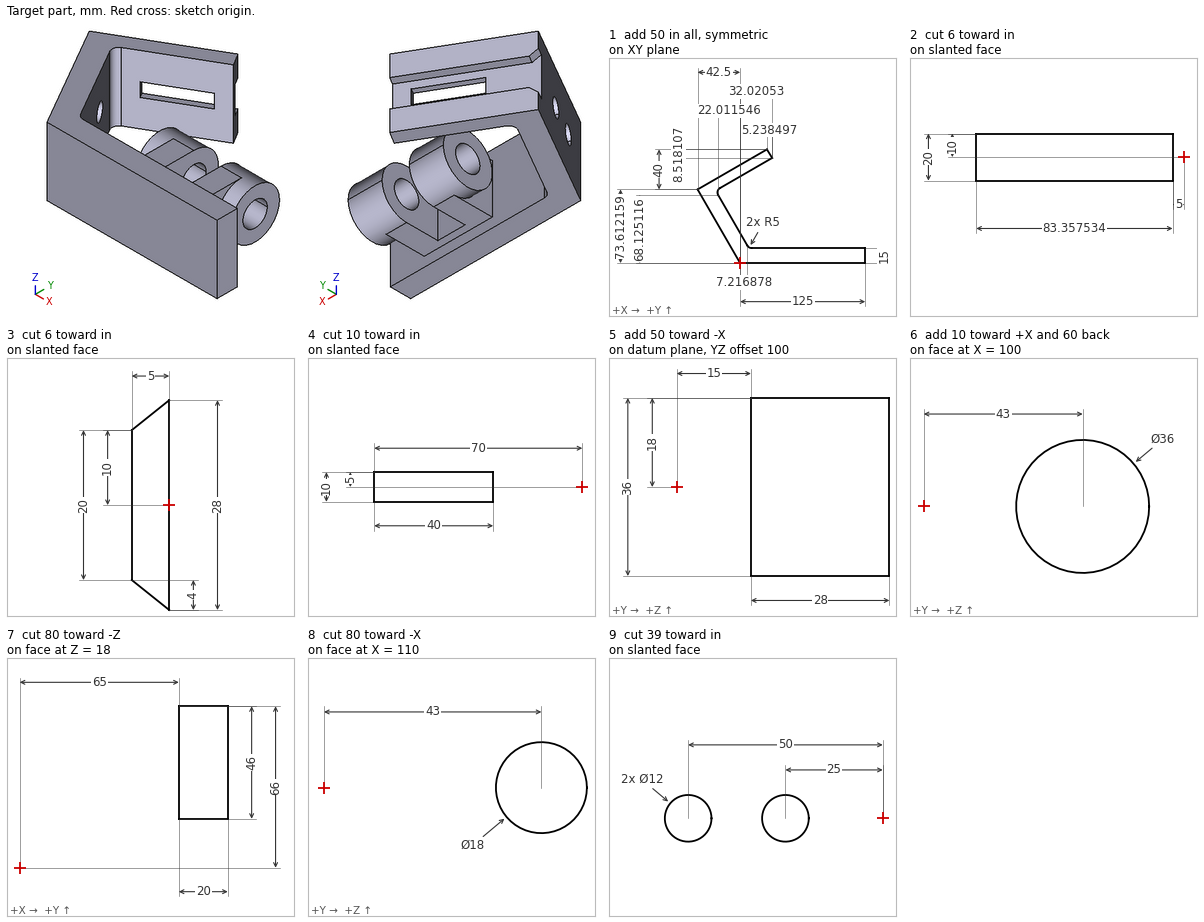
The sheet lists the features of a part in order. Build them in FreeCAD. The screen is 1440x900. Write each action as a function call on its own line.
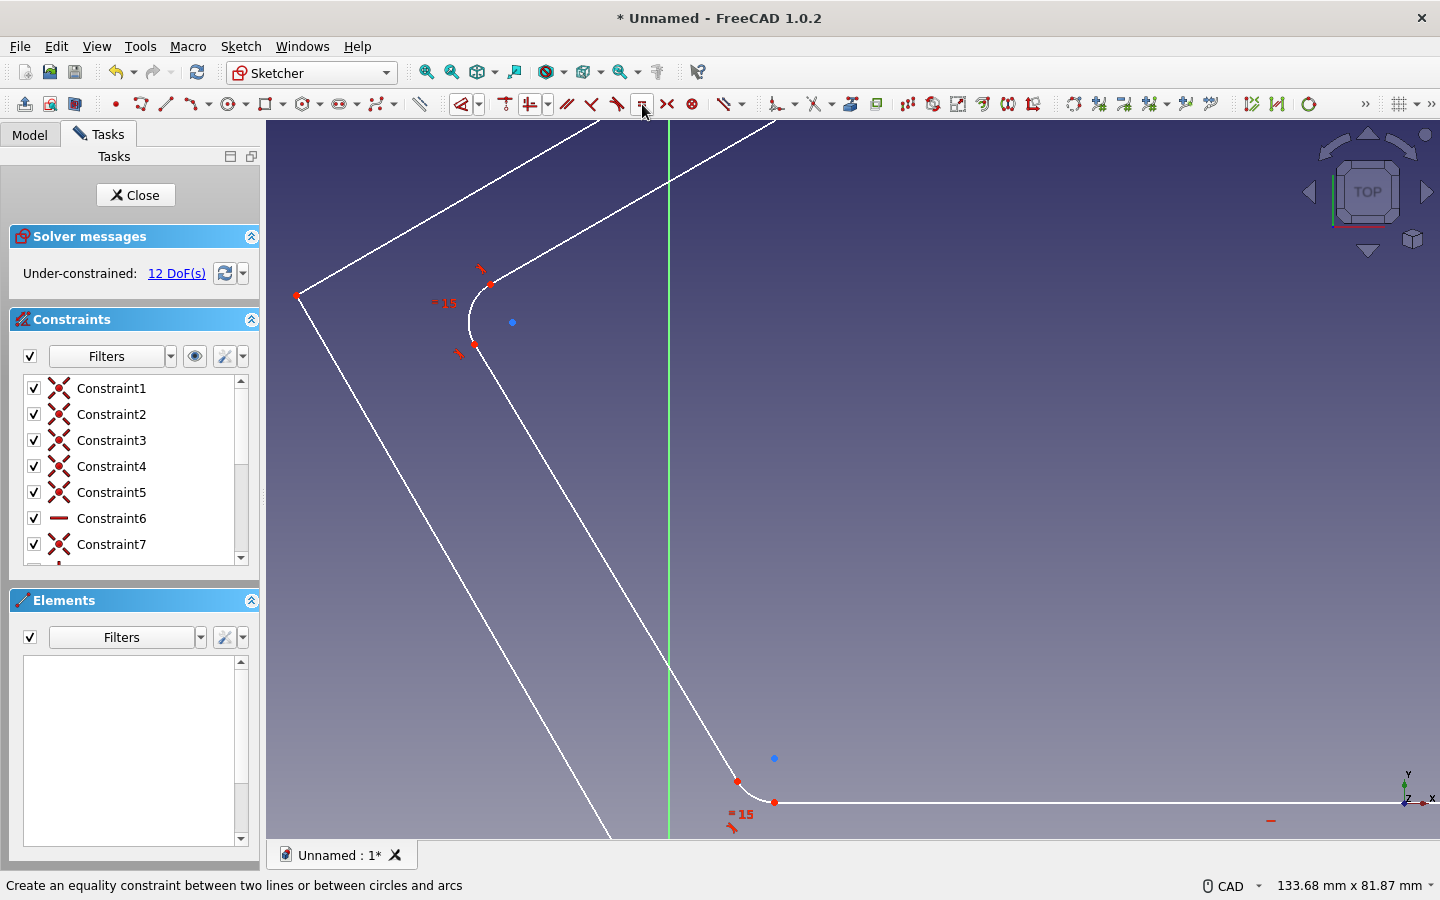
click(460, 104)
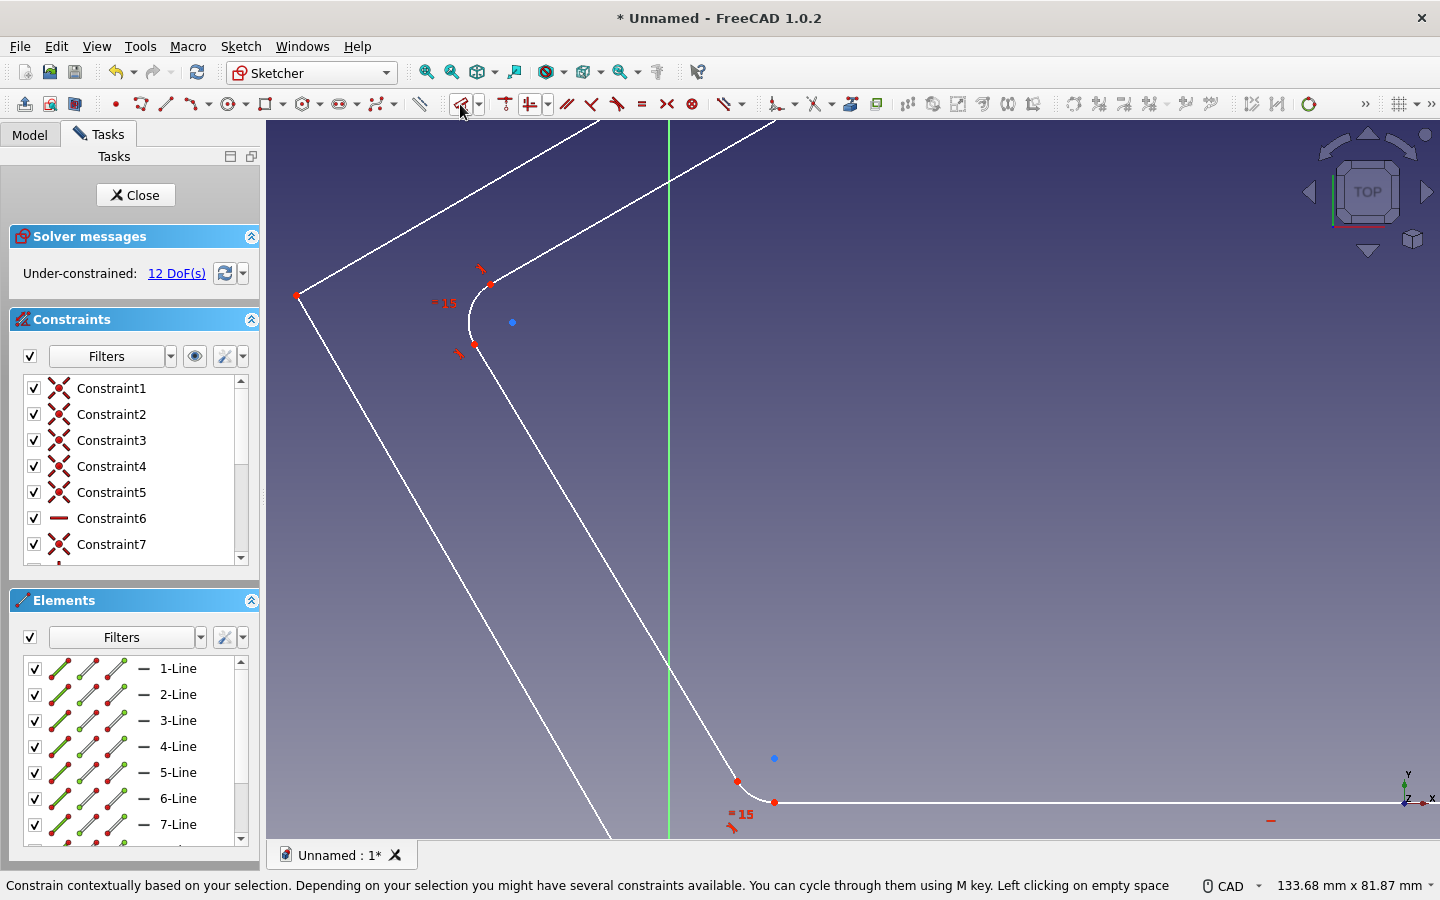
click(476, 299)
click(449, 282)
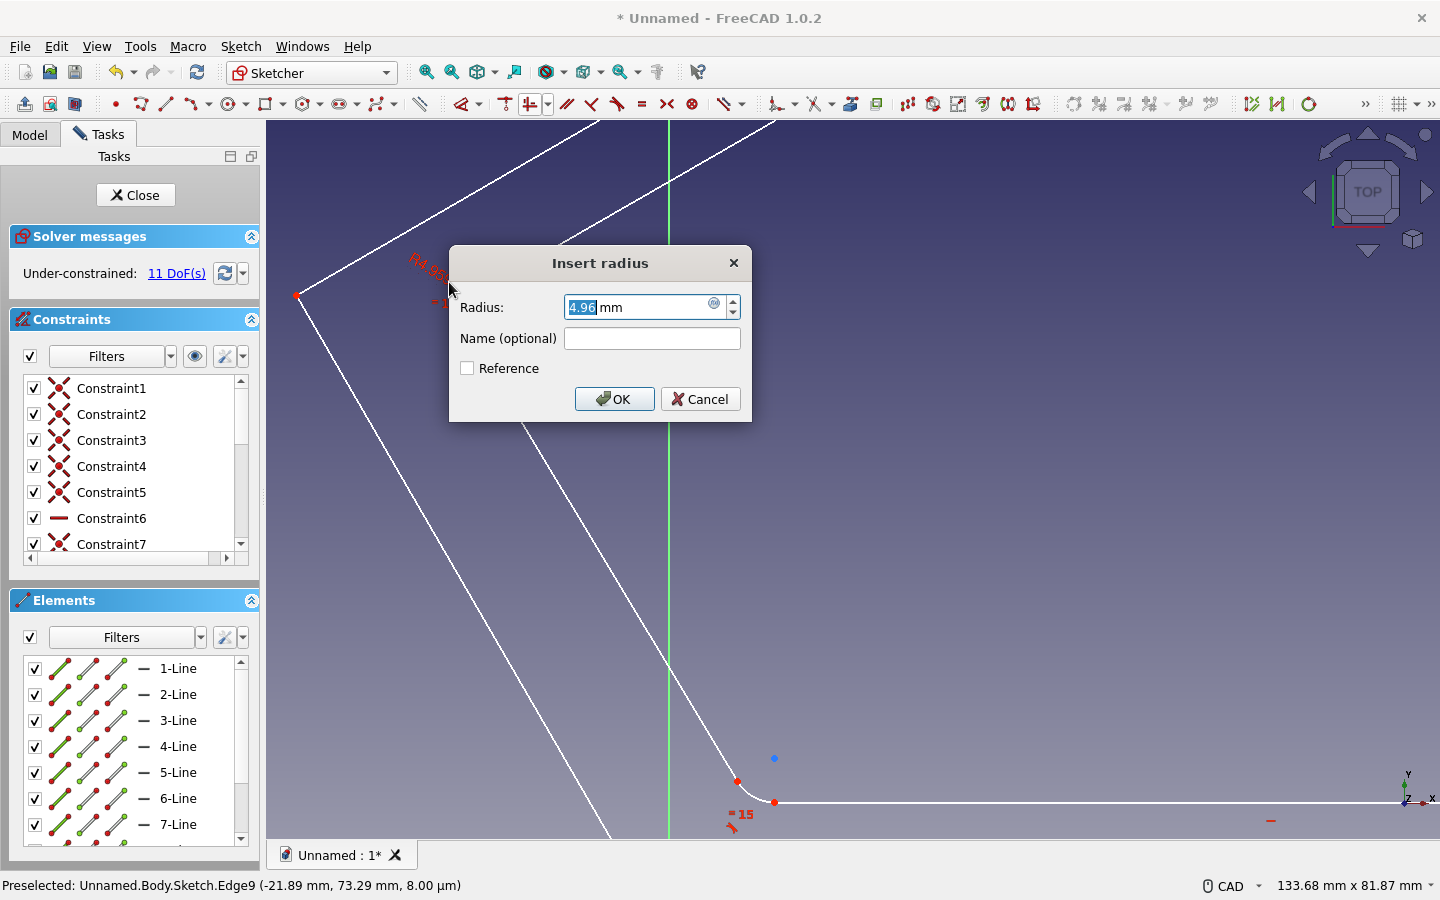
text(5)
key(Return)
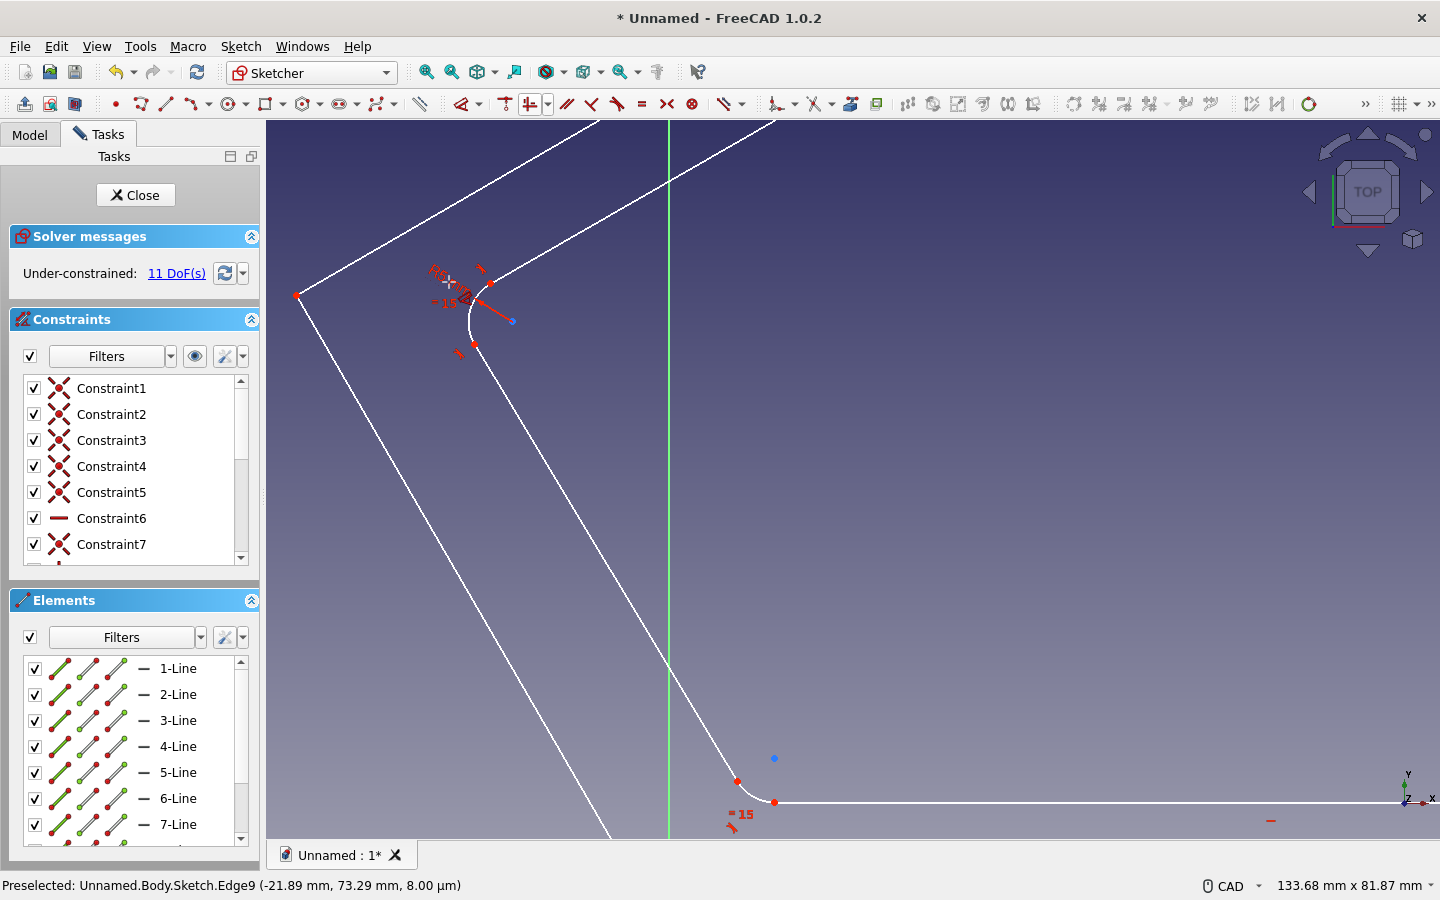
scroll(583, 511, down, 4)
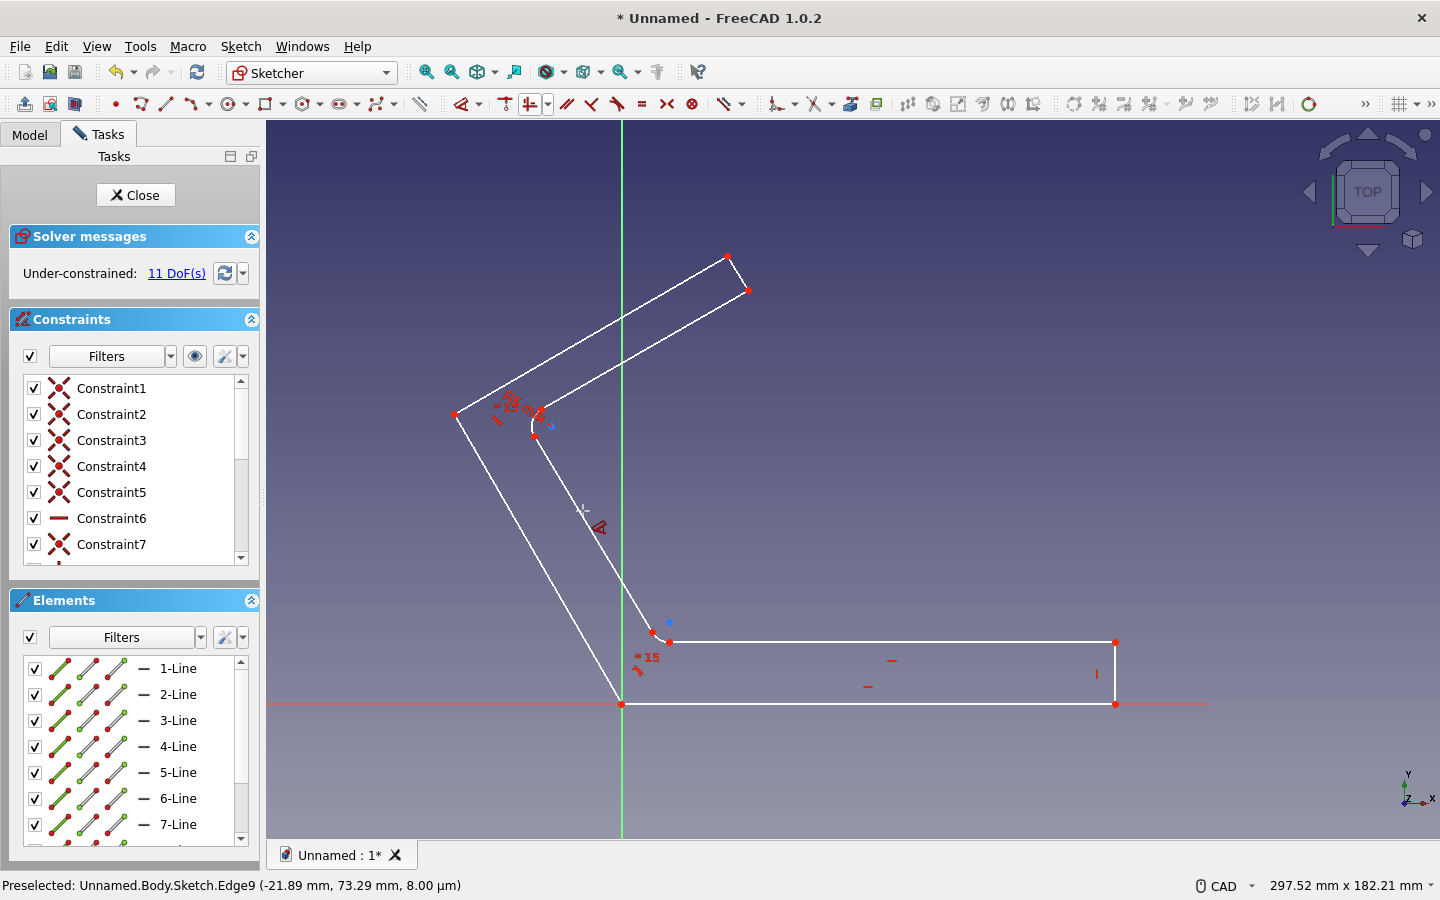
click(1115, 685)
click(1149, 673)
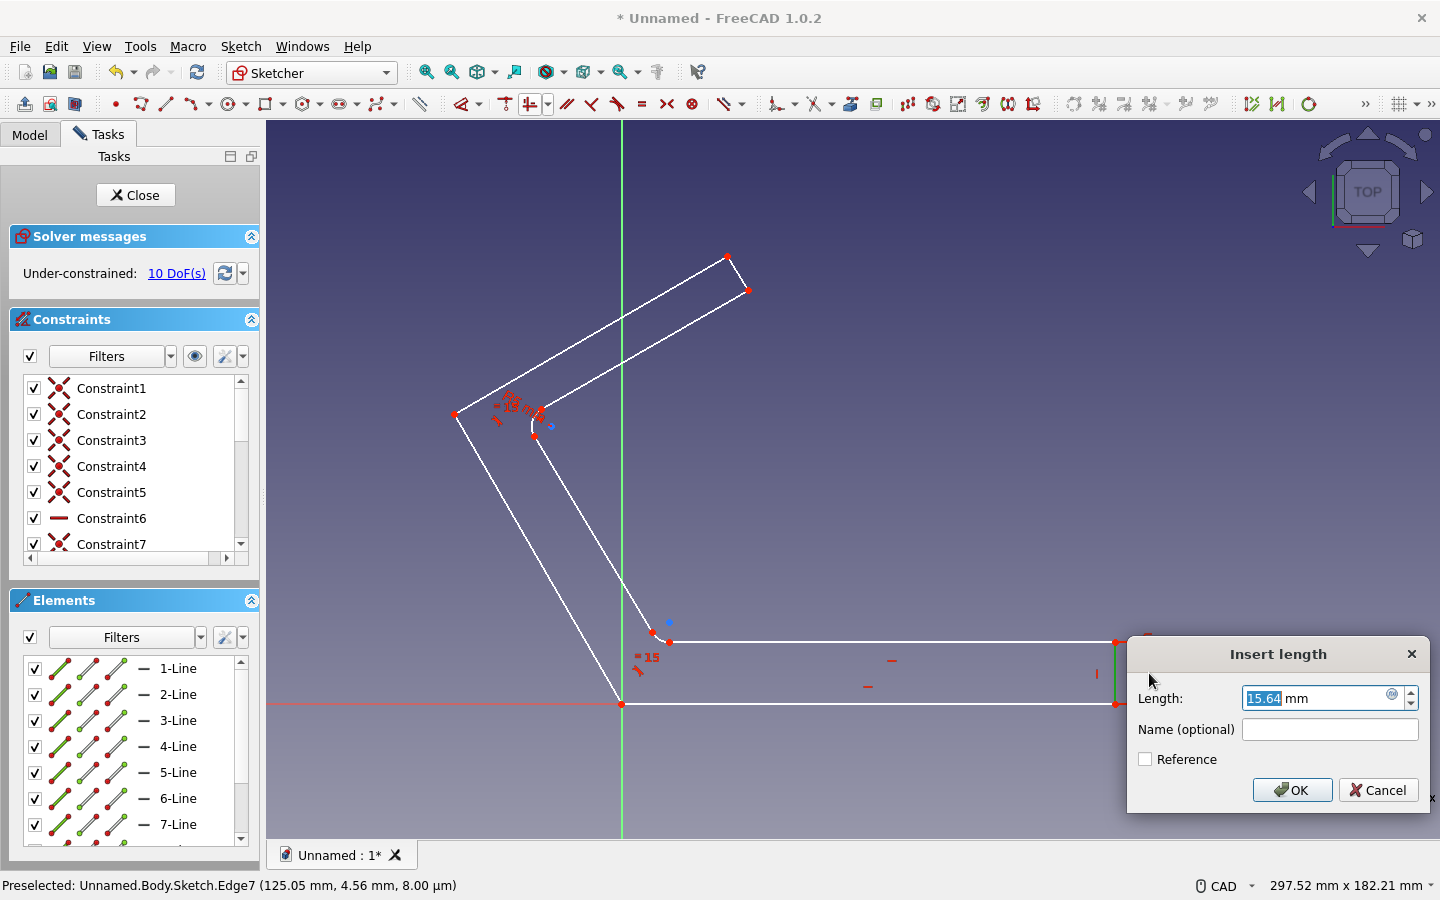
text(15)
key(Return)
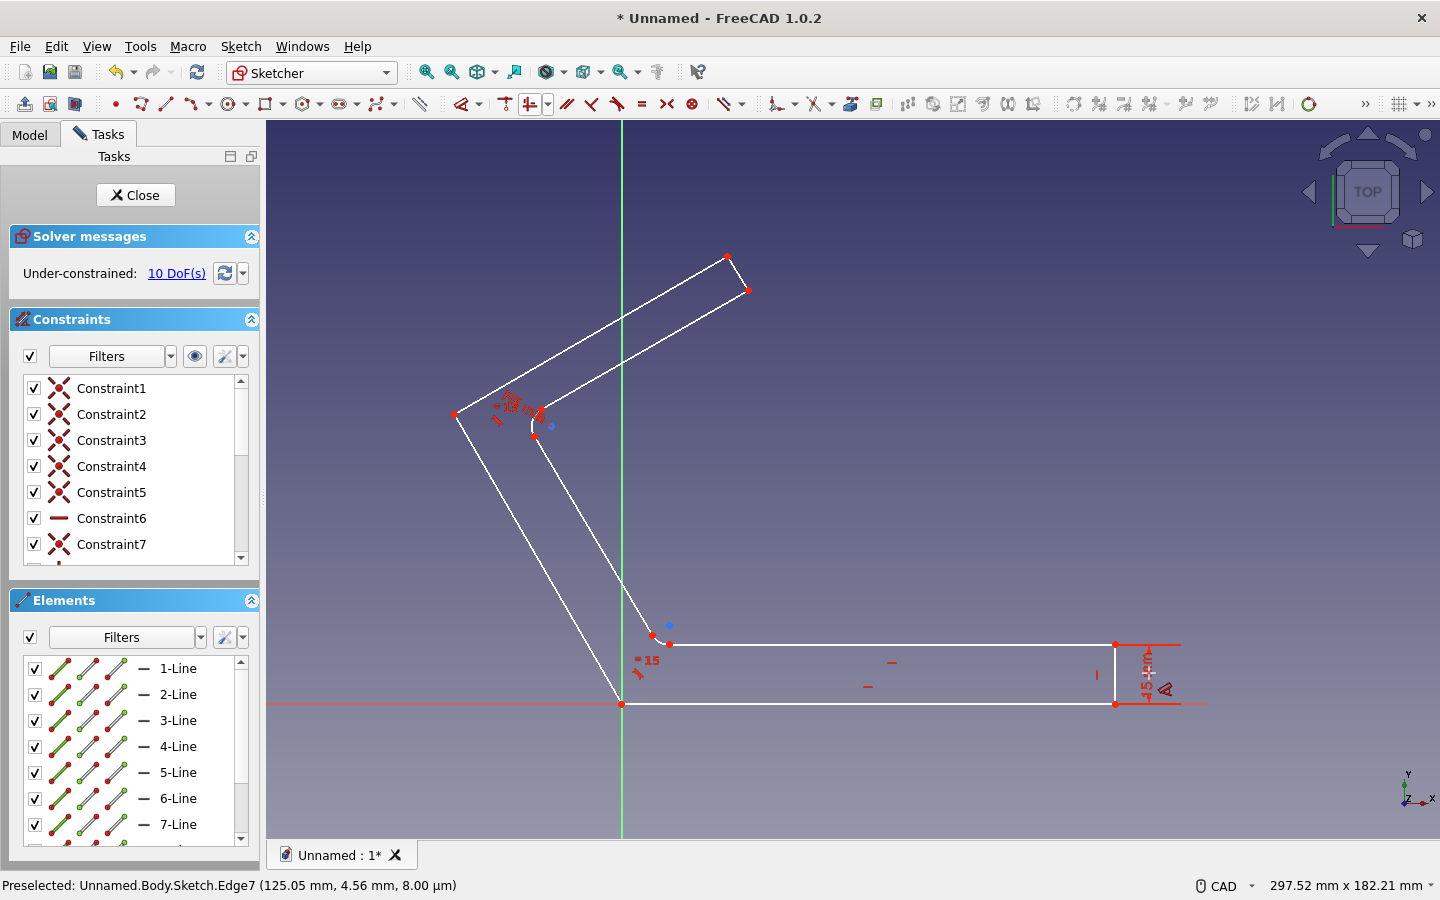
click(770, 704)
click(869, 738)